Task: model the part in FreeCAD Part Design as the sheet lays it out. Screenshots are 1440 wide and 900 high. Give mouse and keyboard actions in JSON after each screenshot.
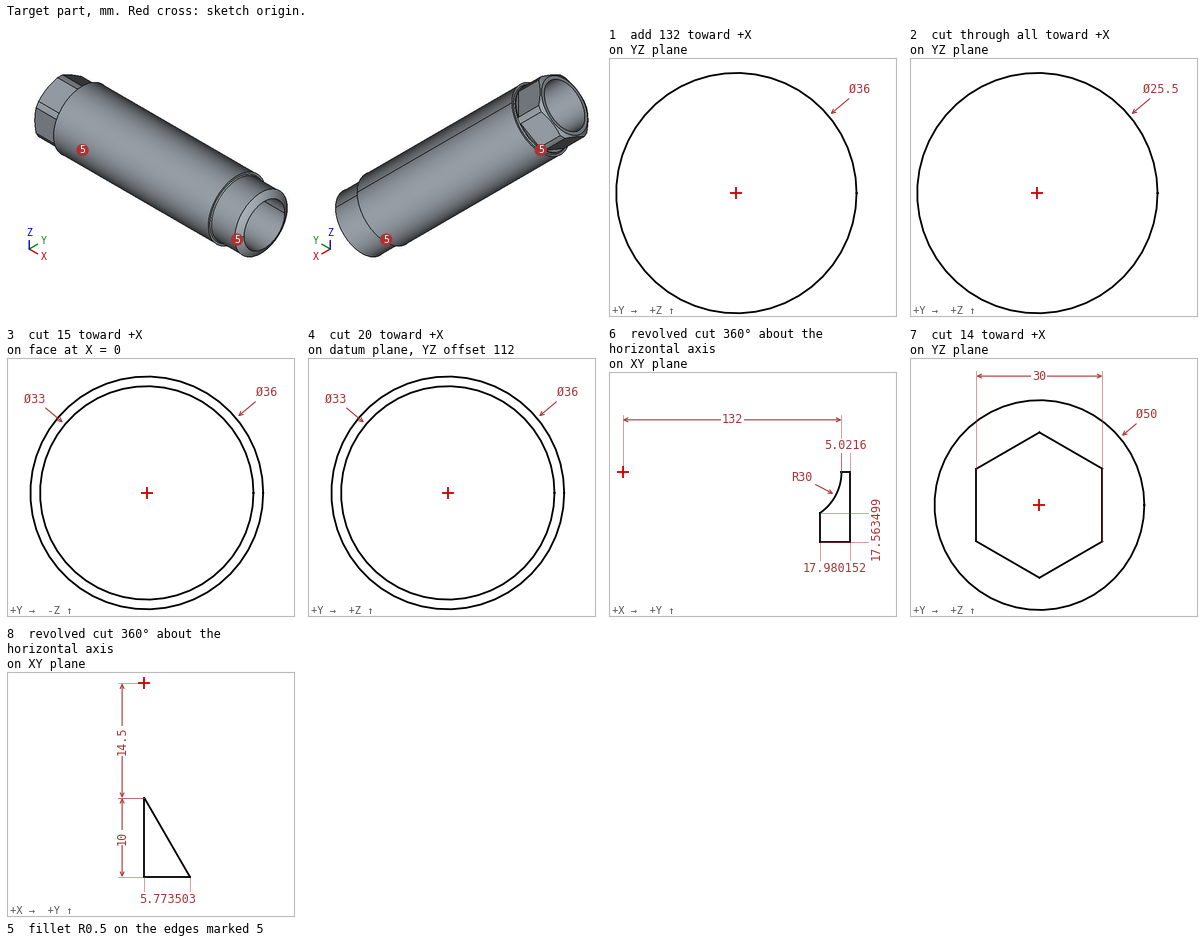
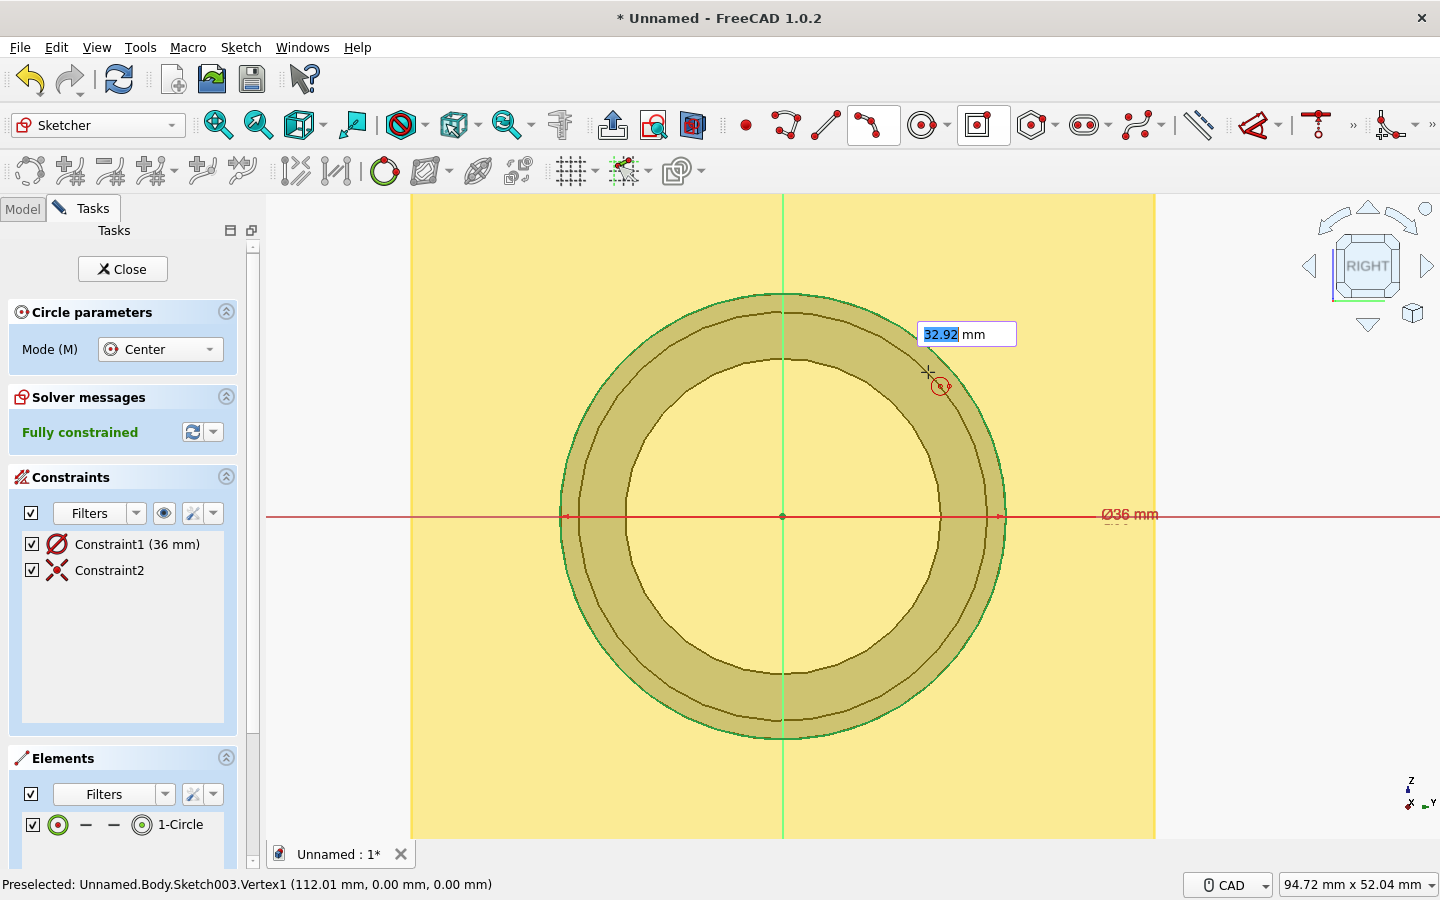
{"action": "type", "text": "33"}
{"action": "key", "text": "Return"}
{"action": "key", "text": "Escape"}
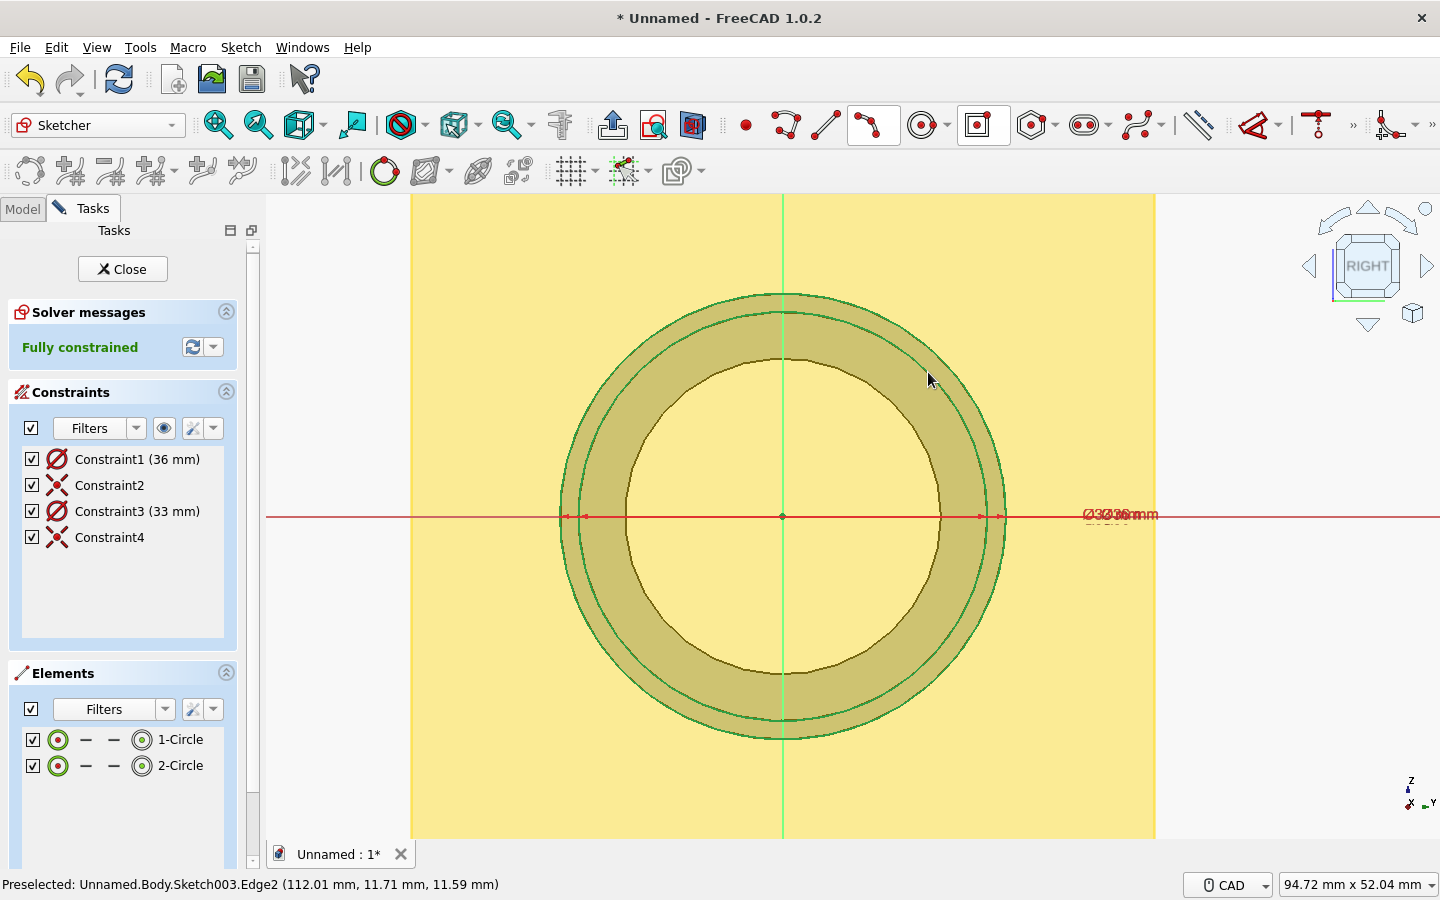
{"action": "left_click", "coordinate": [123, 269]}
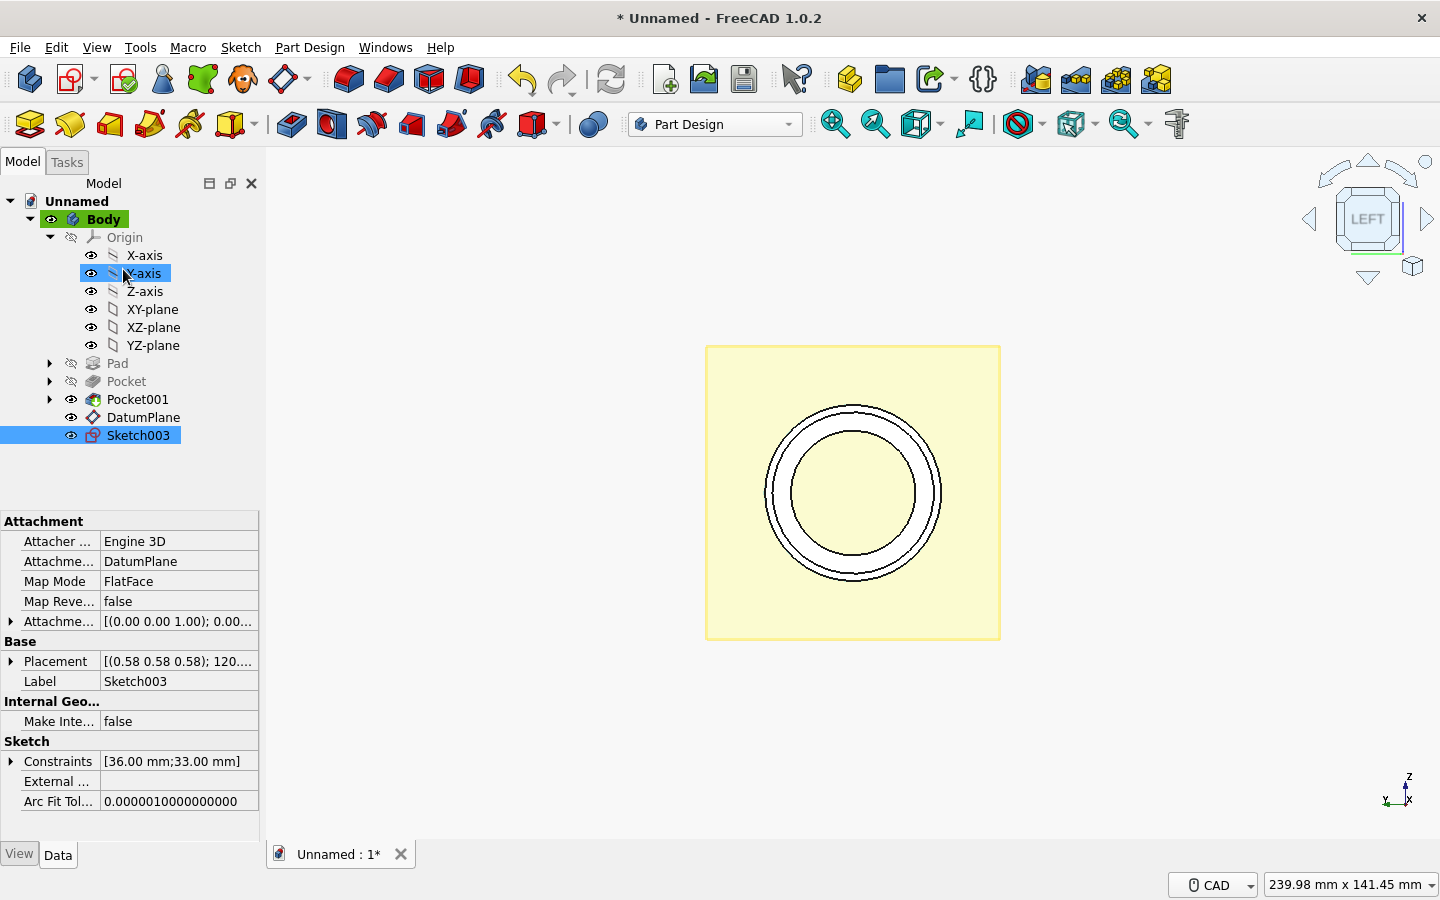
{"action": "left_click", "coordinate": [292, 124]}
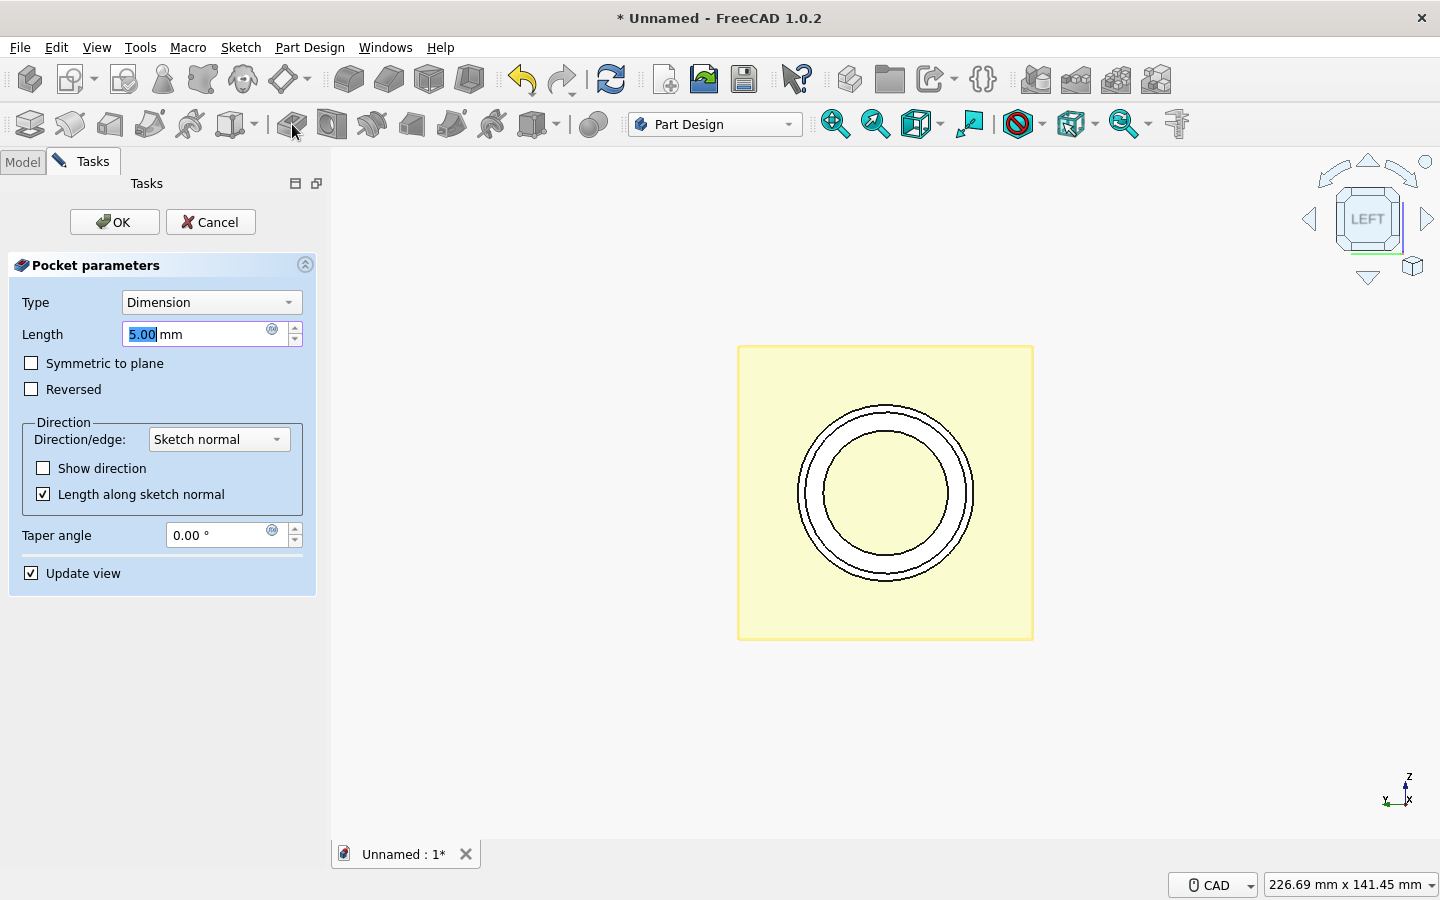
{"action": "type", "text": "20"}
{"action": "key", "text": "Tab"}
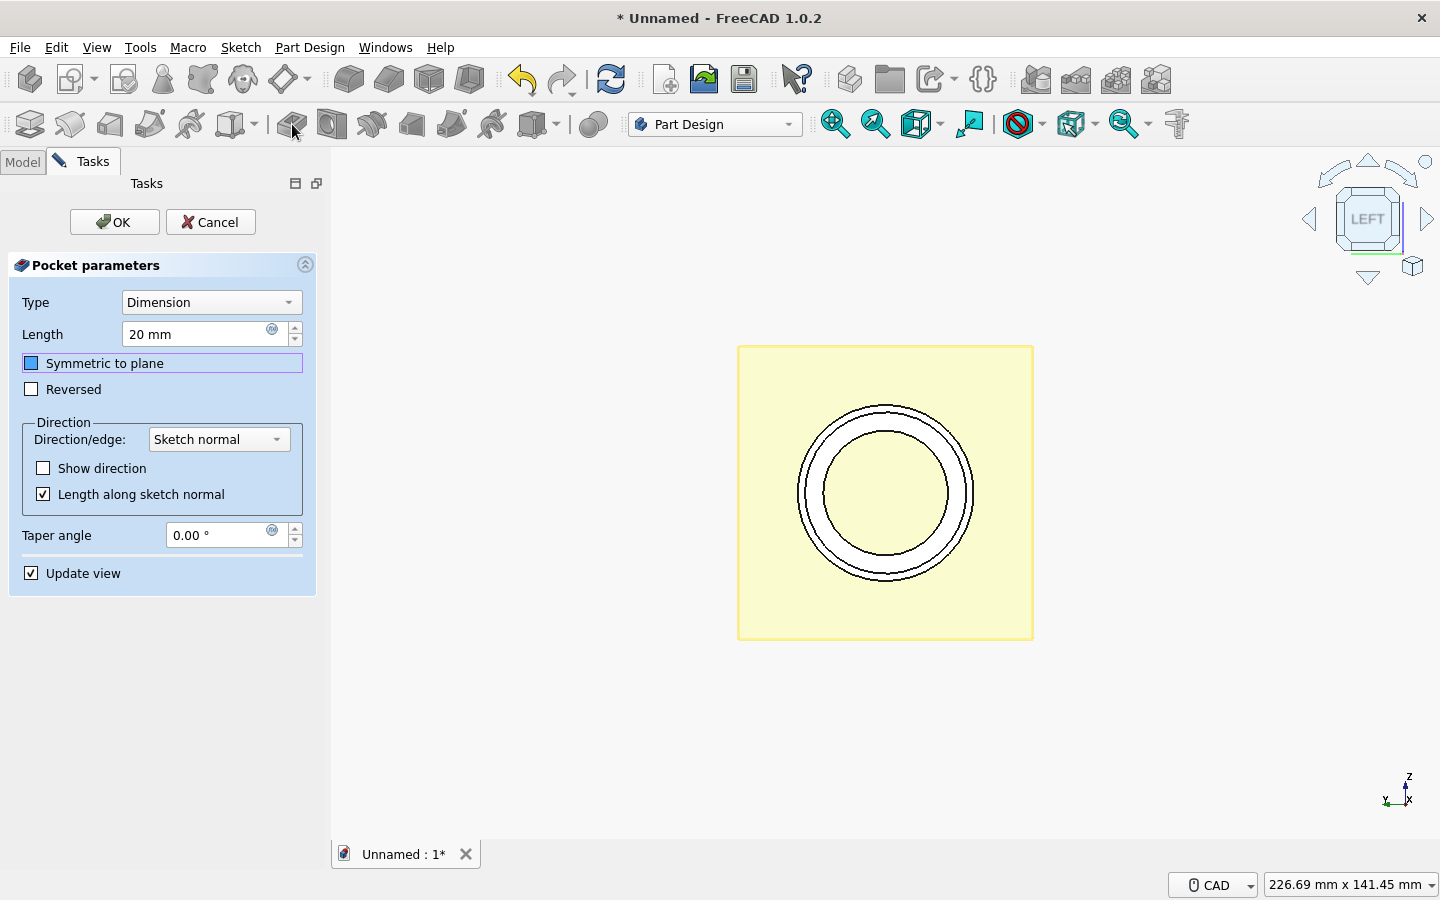
{"action": "left_click", "coordinate": [30, 389]}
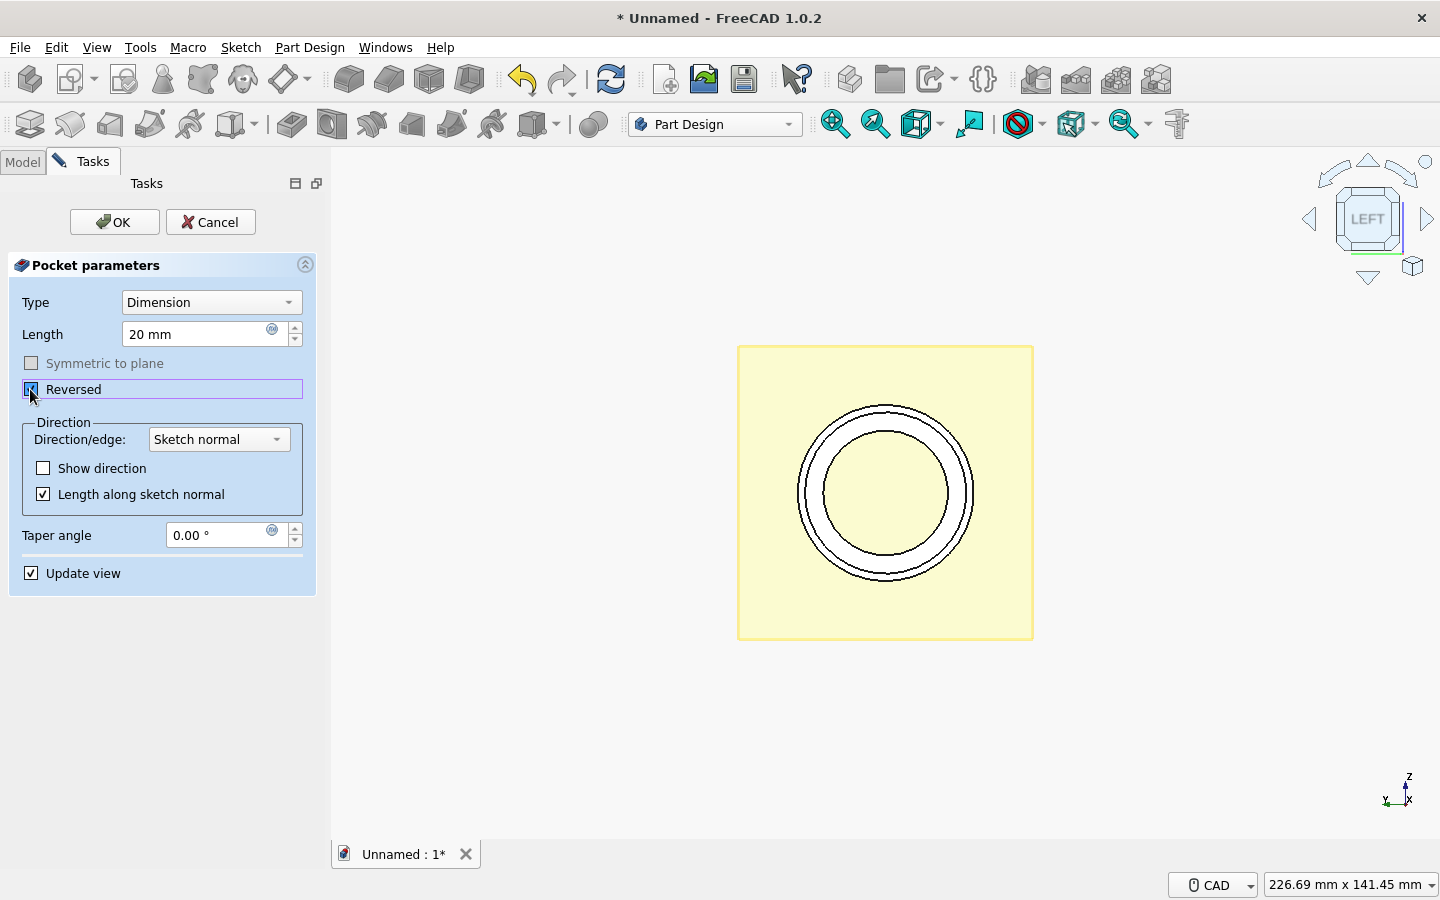
{"action": "left_click", "coordinate": [115, 222]}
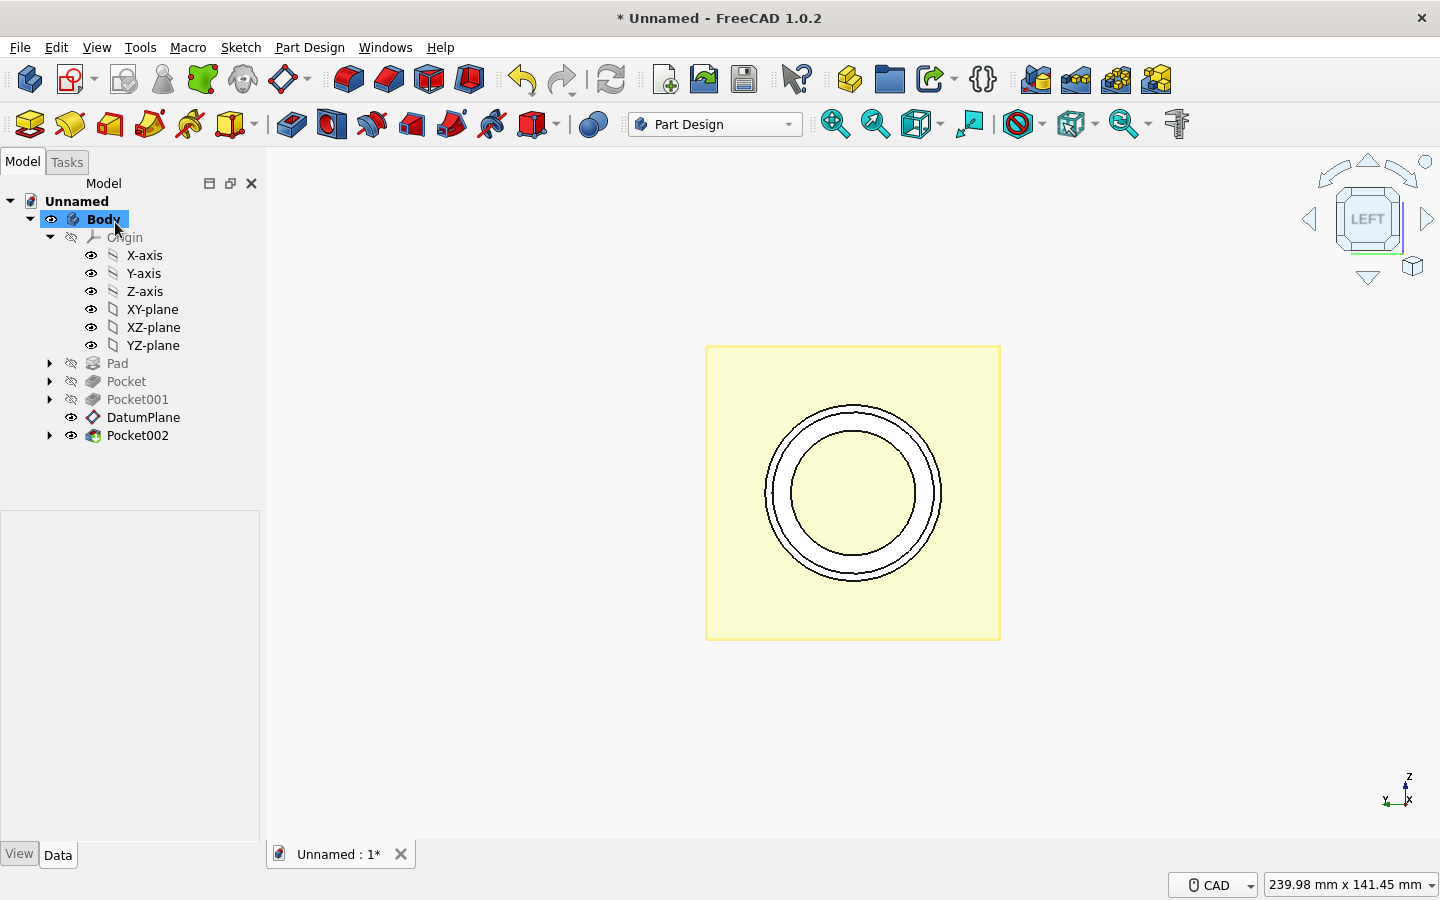
{"action": "left_click", "coordinate": [116, 417]}
{"action": "key", "text": "space"}